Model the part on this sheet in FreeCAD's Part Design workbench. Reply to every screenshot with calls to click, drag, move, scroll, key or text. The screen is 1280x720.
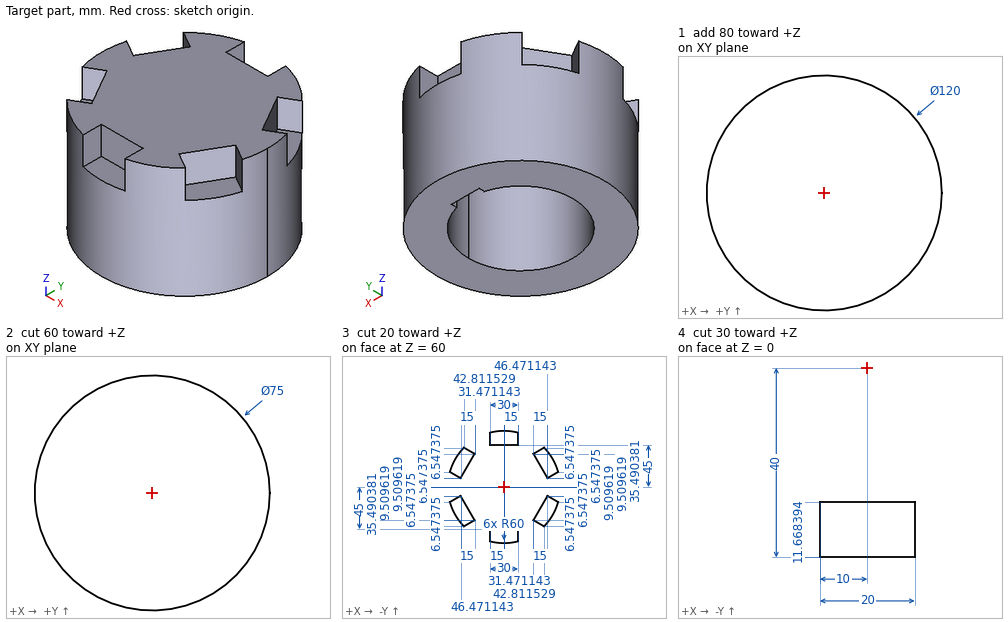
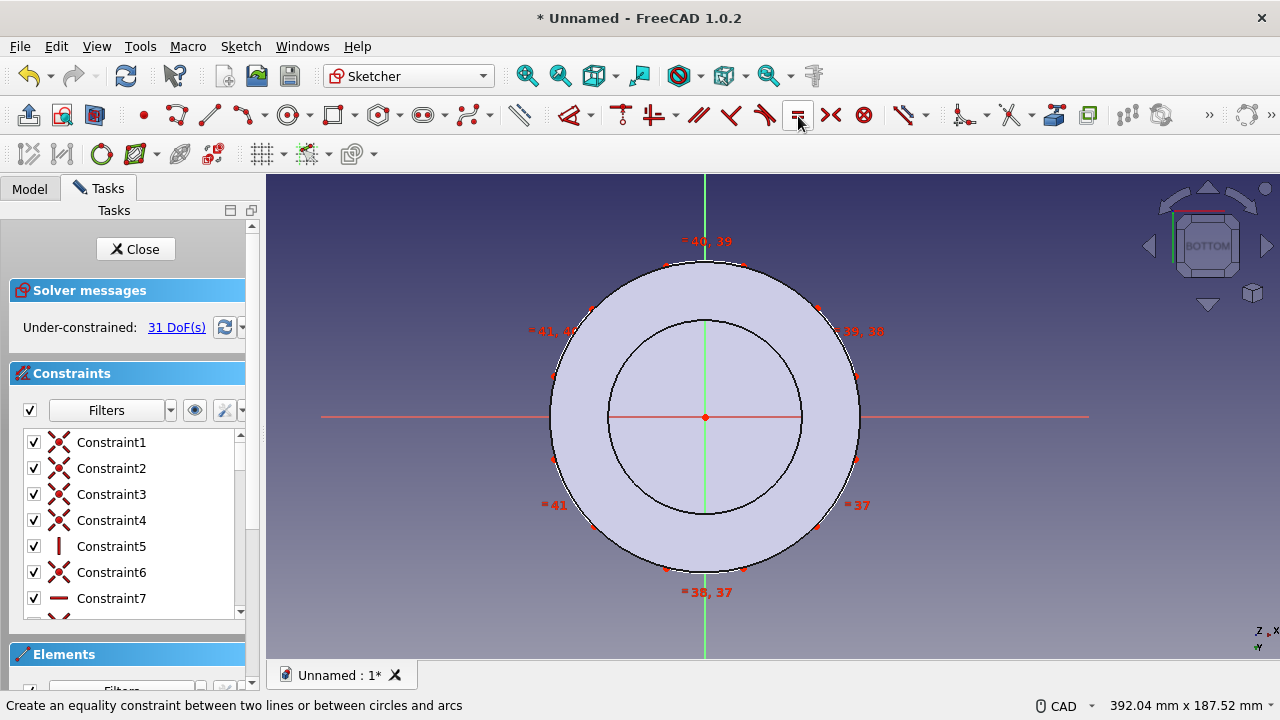
click(568, 116)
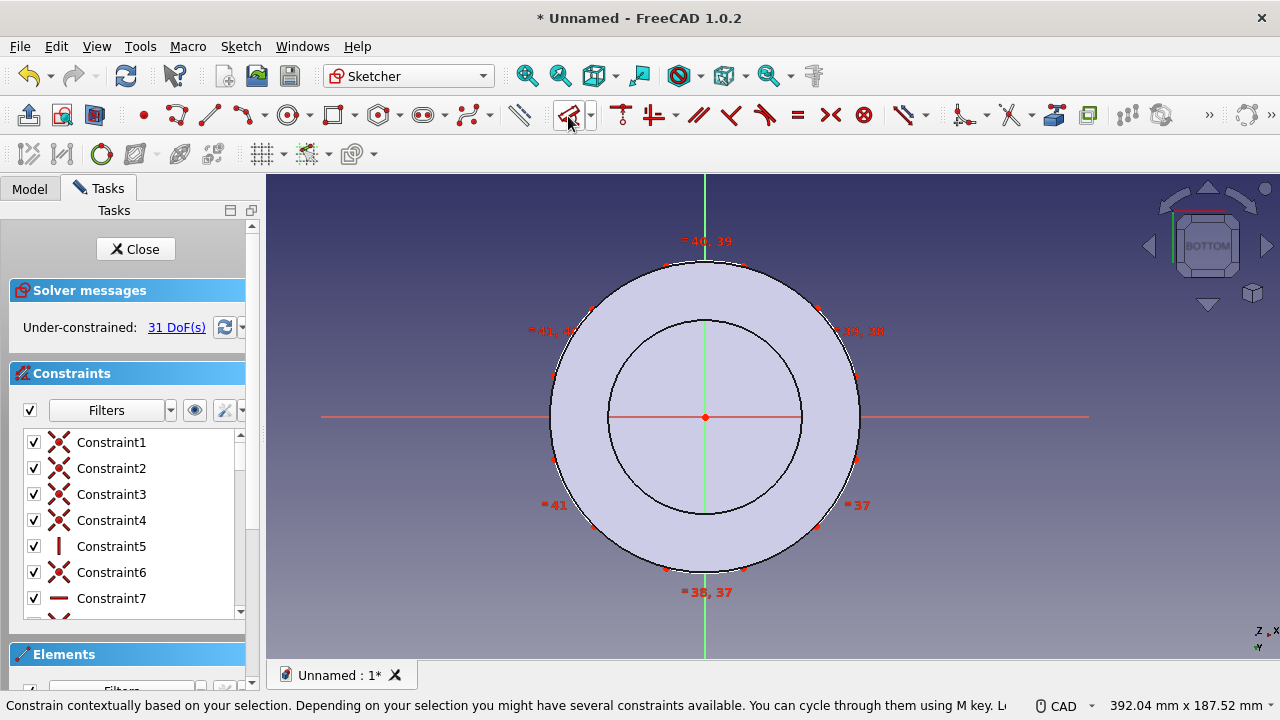
click(831, 509)
click(857, 528)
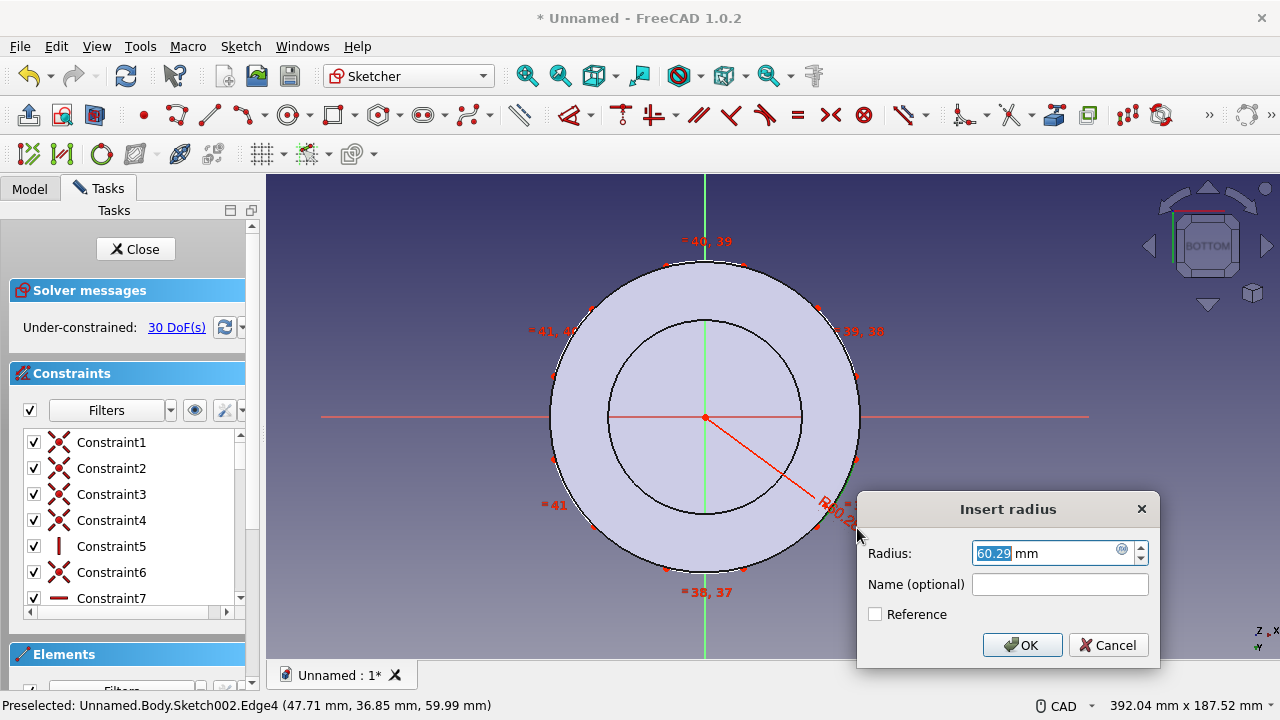
text(60)
key(Return)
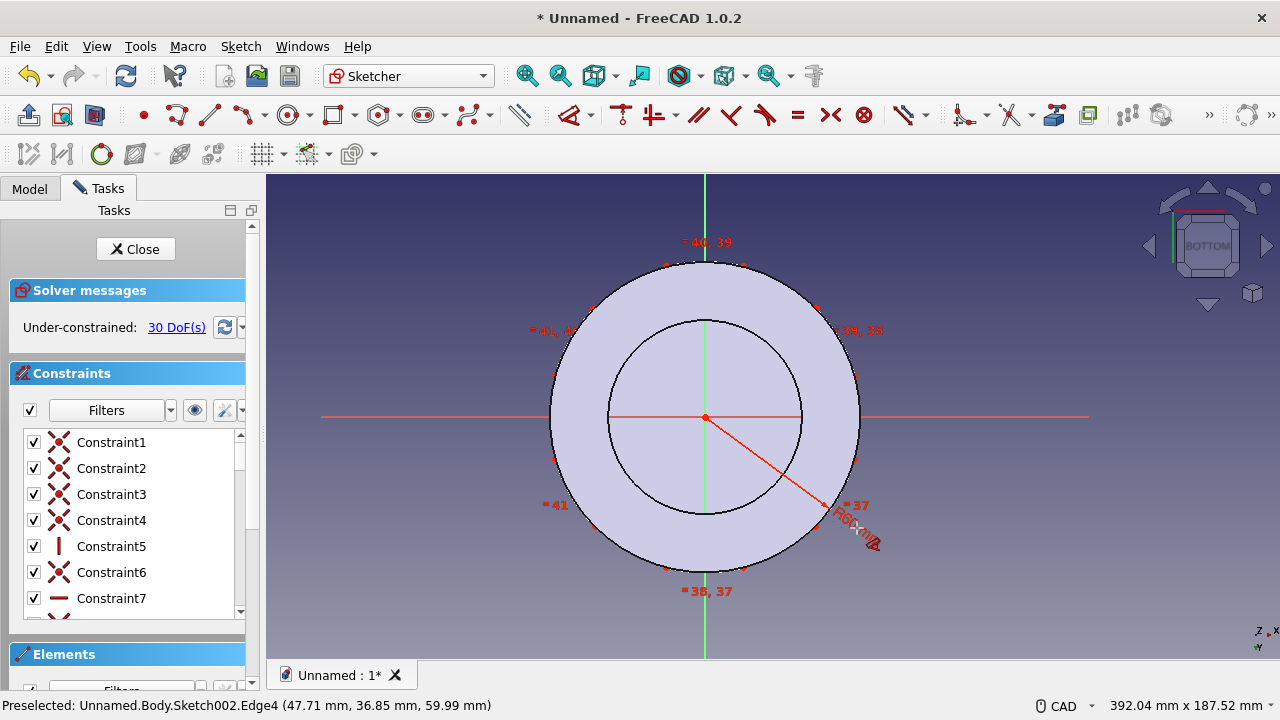
click(689, 535)
click(687, 501)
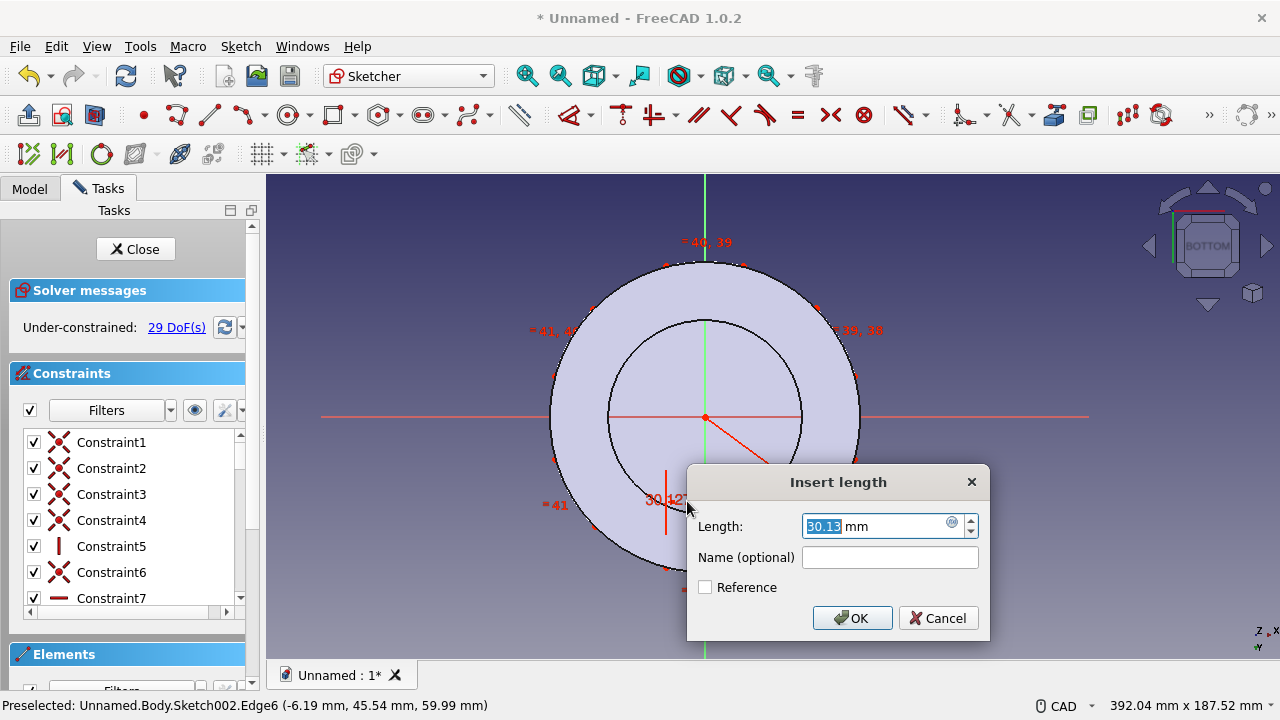
text(30)
key(Return)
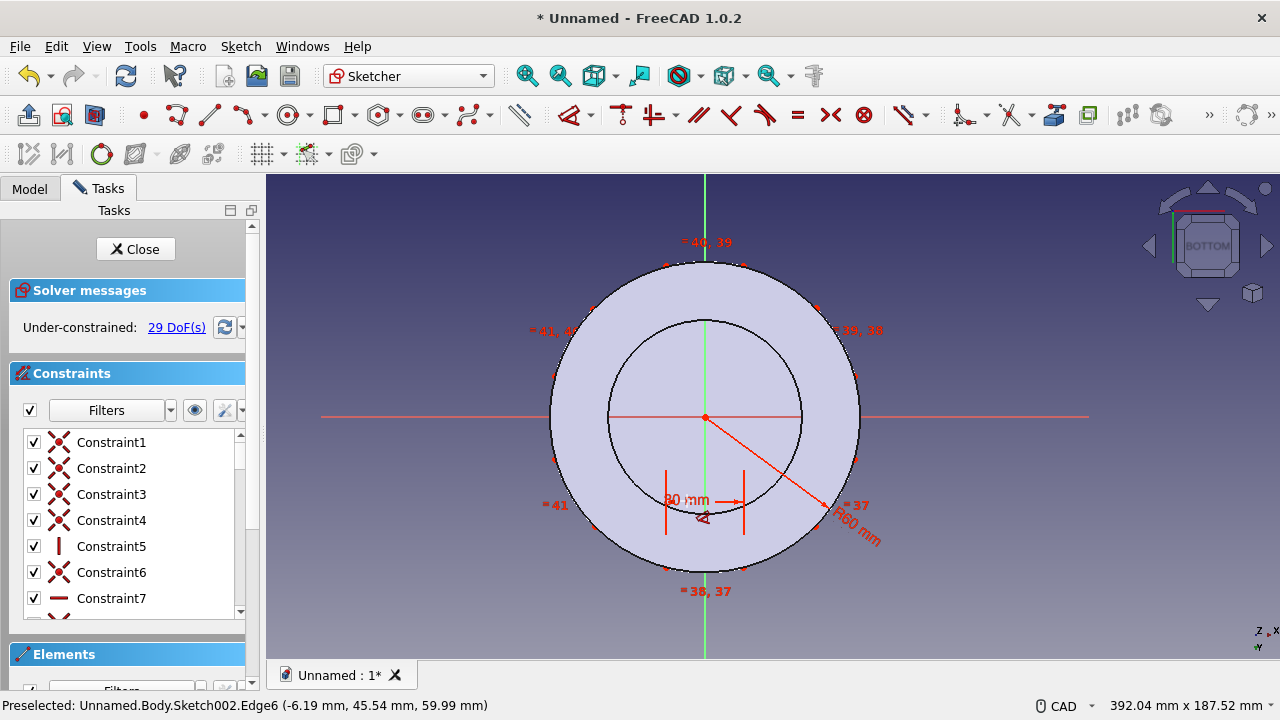
click(721, 302)
click(687, 336)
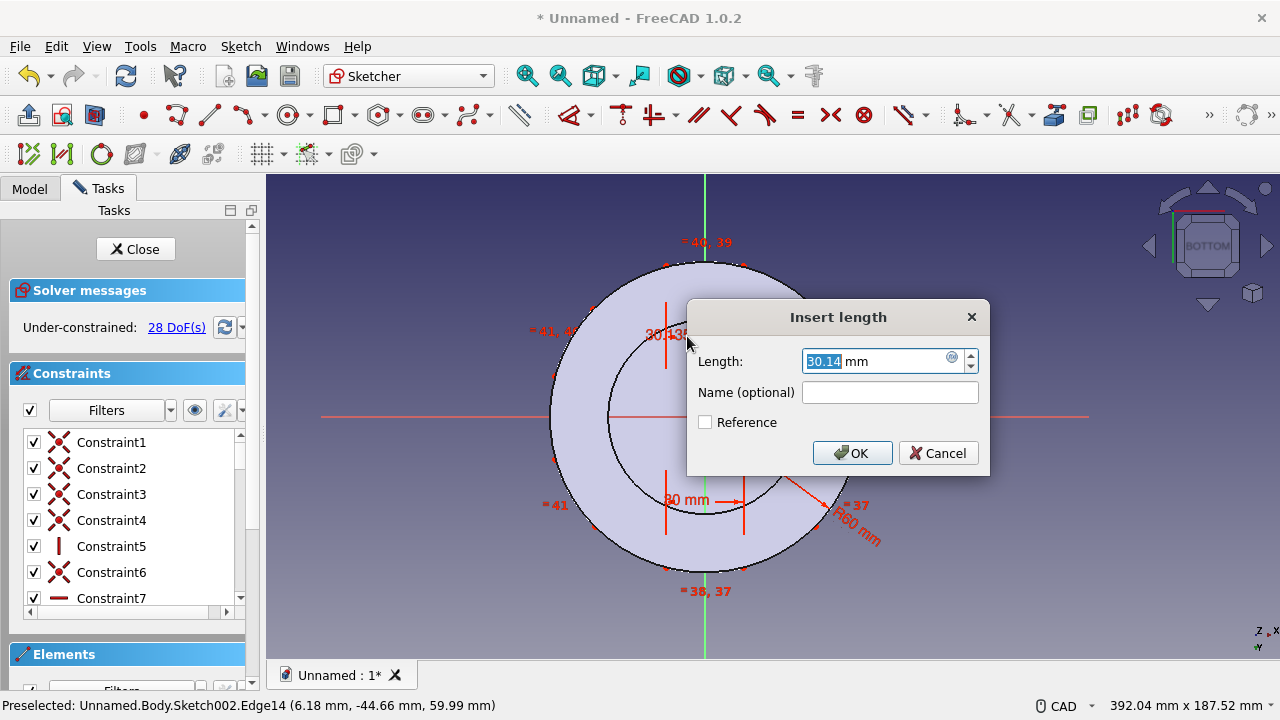
text(30)
key(Return)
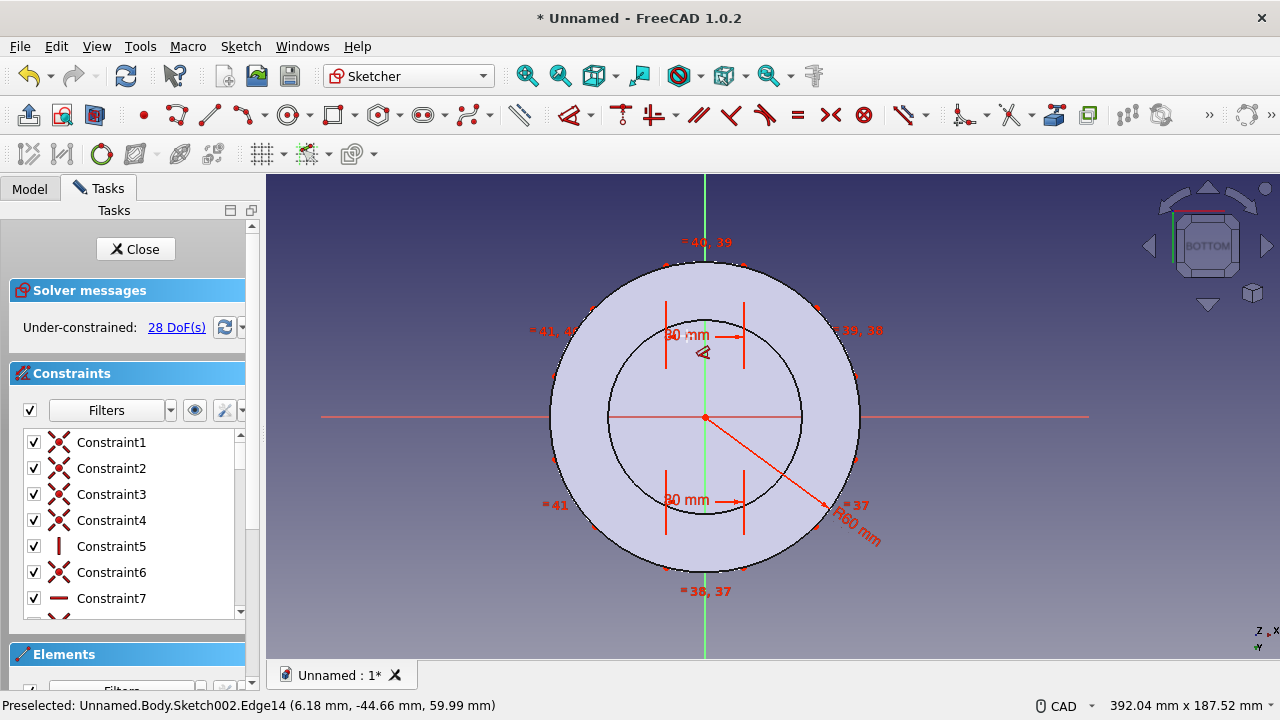
click(666, 567)
click(686, 601)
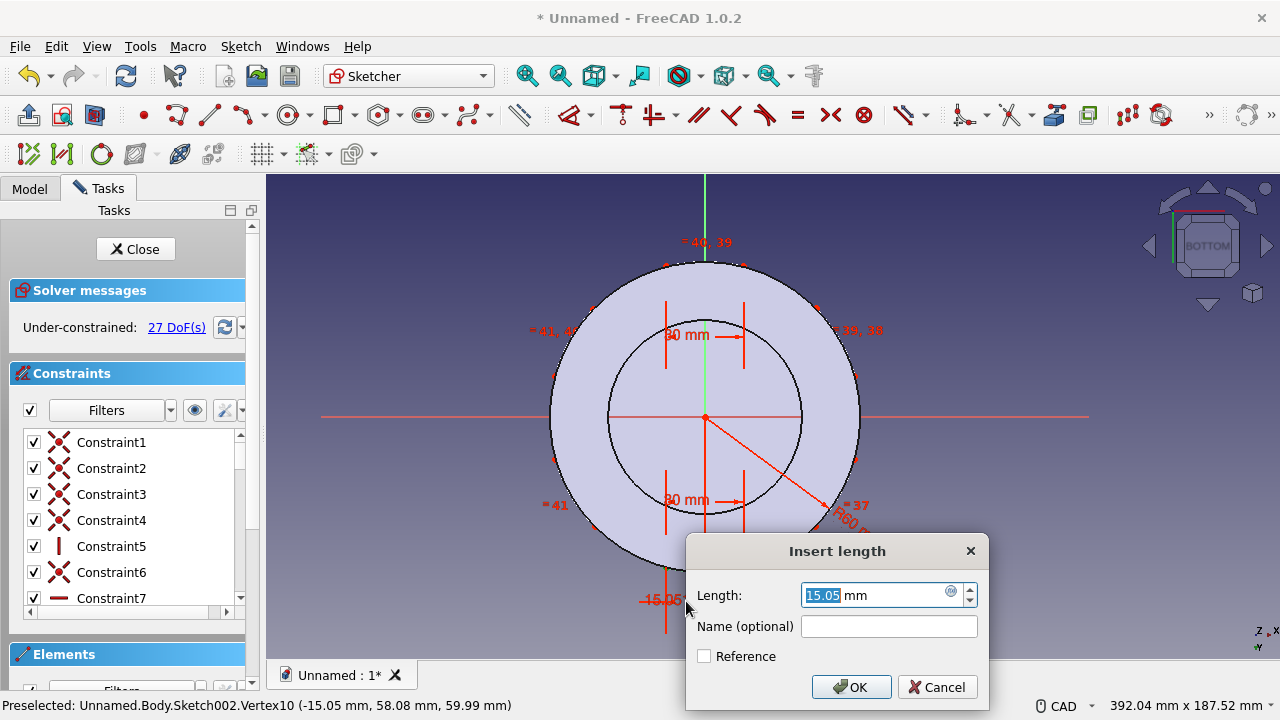
text(15)
key(Return)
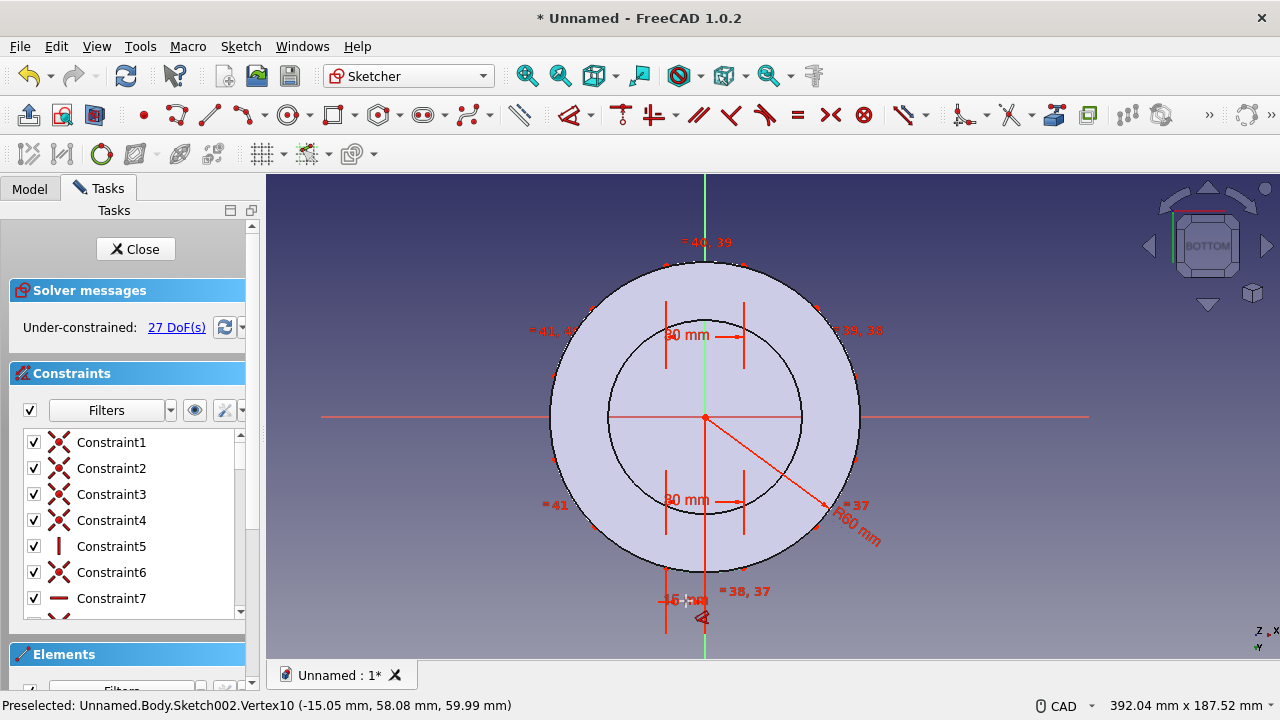
click(666, 535)
click(632, 476)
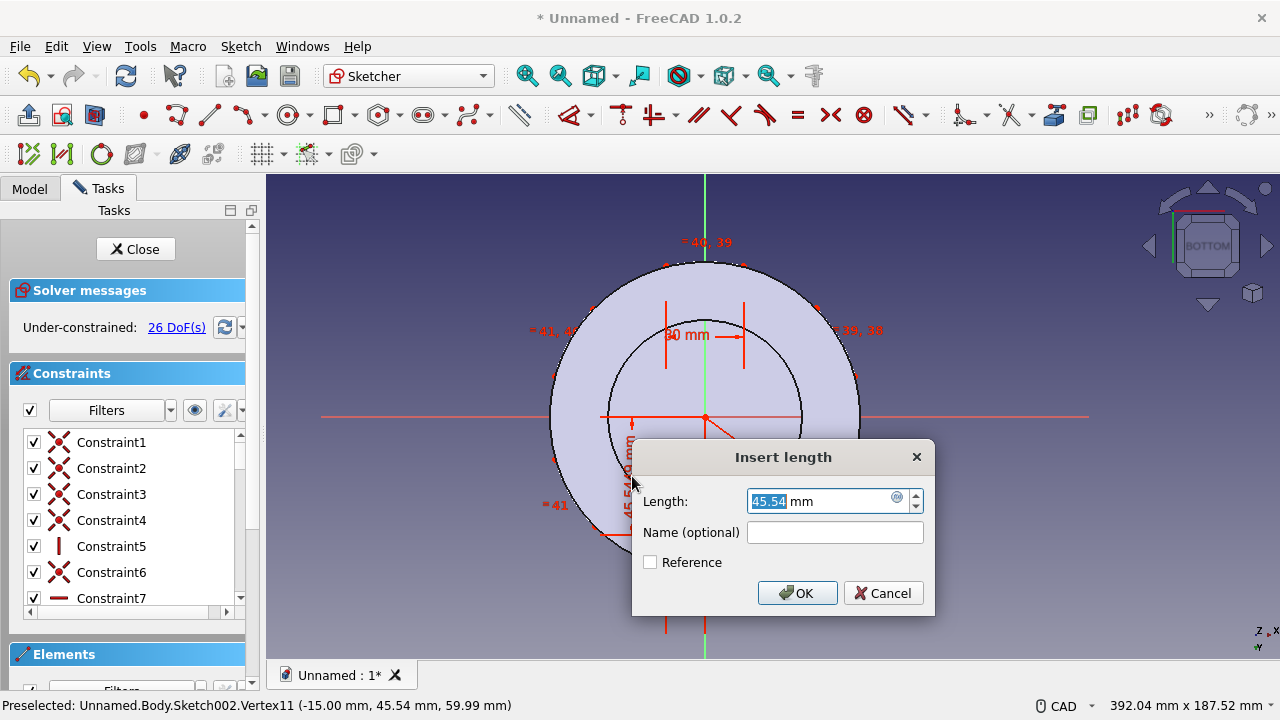
text(45)
key(Return)